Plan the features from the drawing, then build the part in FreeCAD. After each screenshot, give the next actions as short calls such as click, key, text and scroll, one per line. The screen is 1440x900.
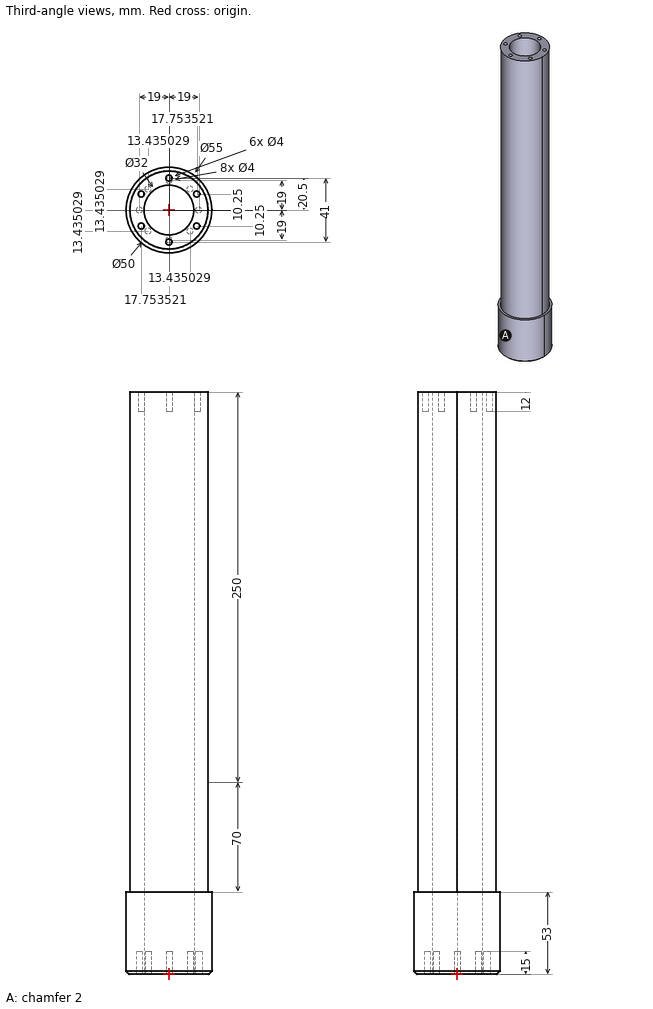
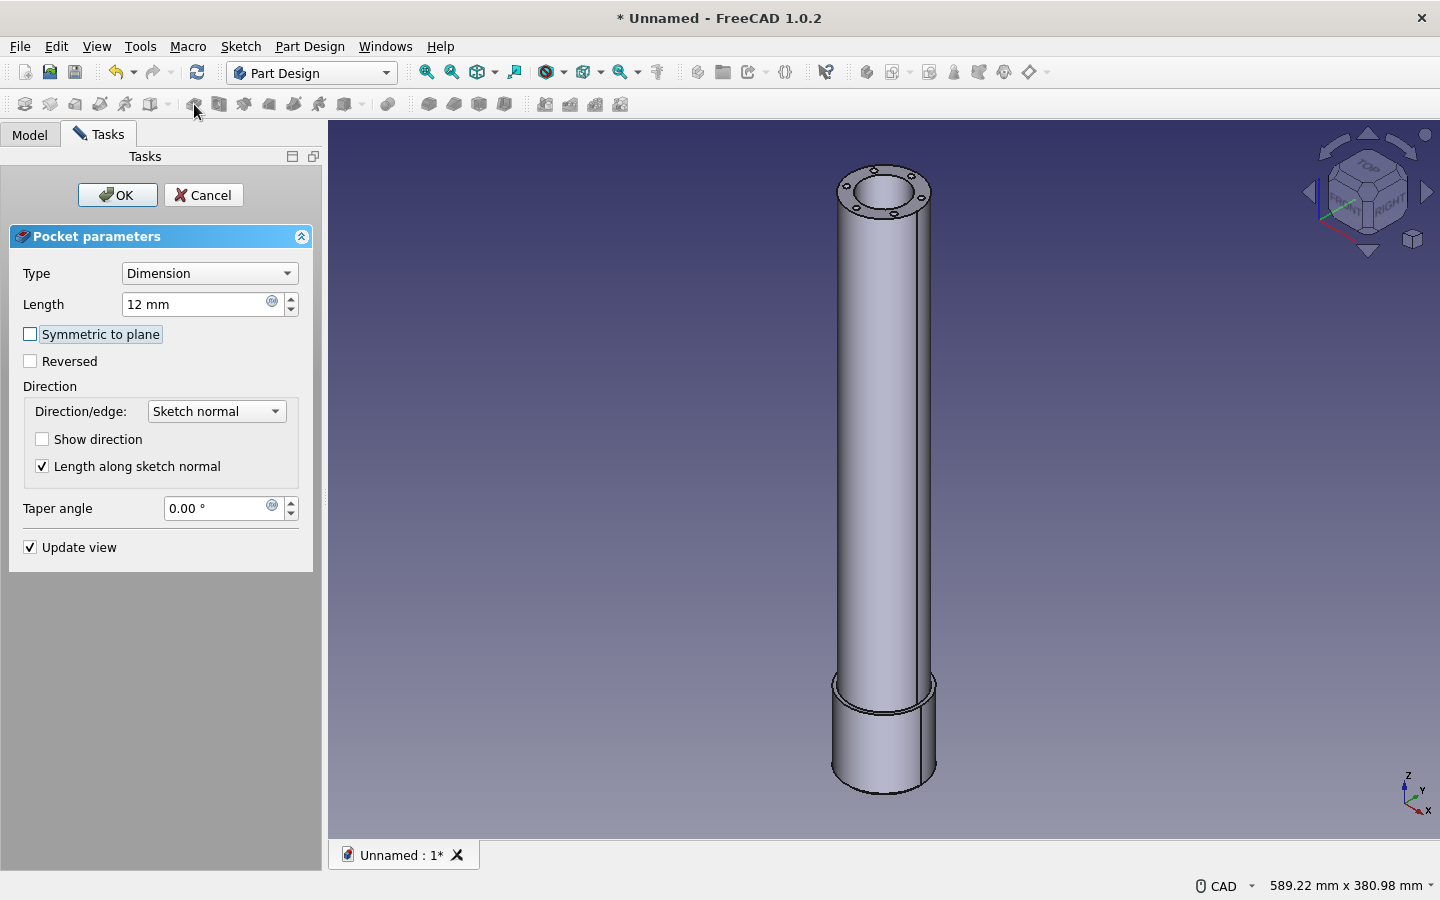
click(118, 195)